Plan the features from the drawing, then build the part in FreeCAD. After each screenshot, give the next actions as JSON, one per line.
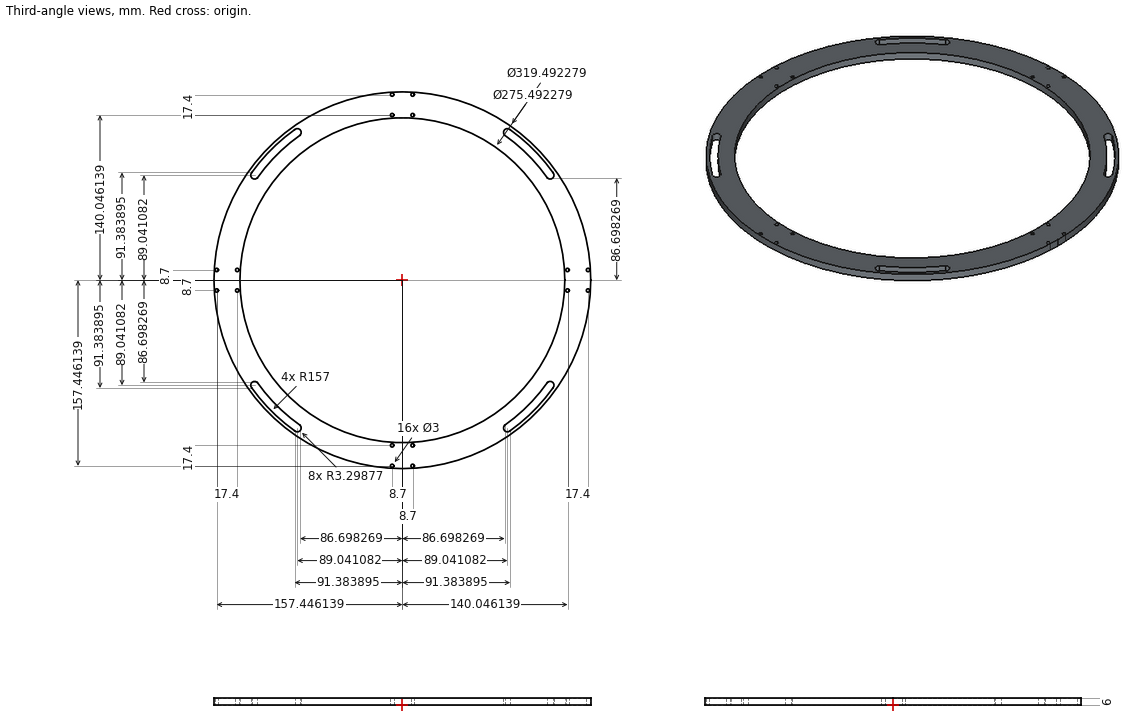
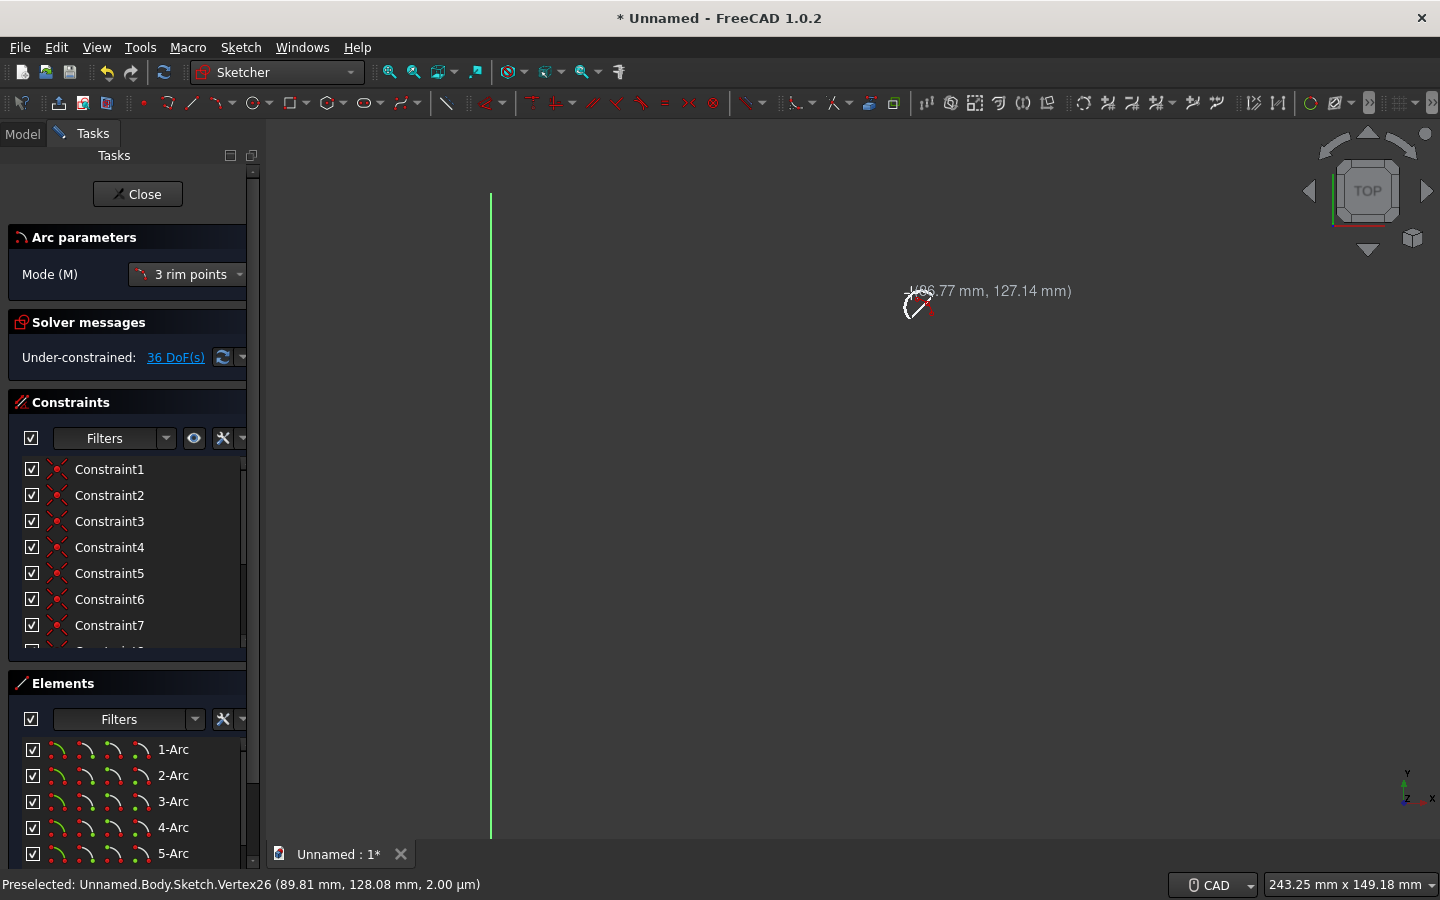
{"action": "left_click", "coordinate": [909, 293]}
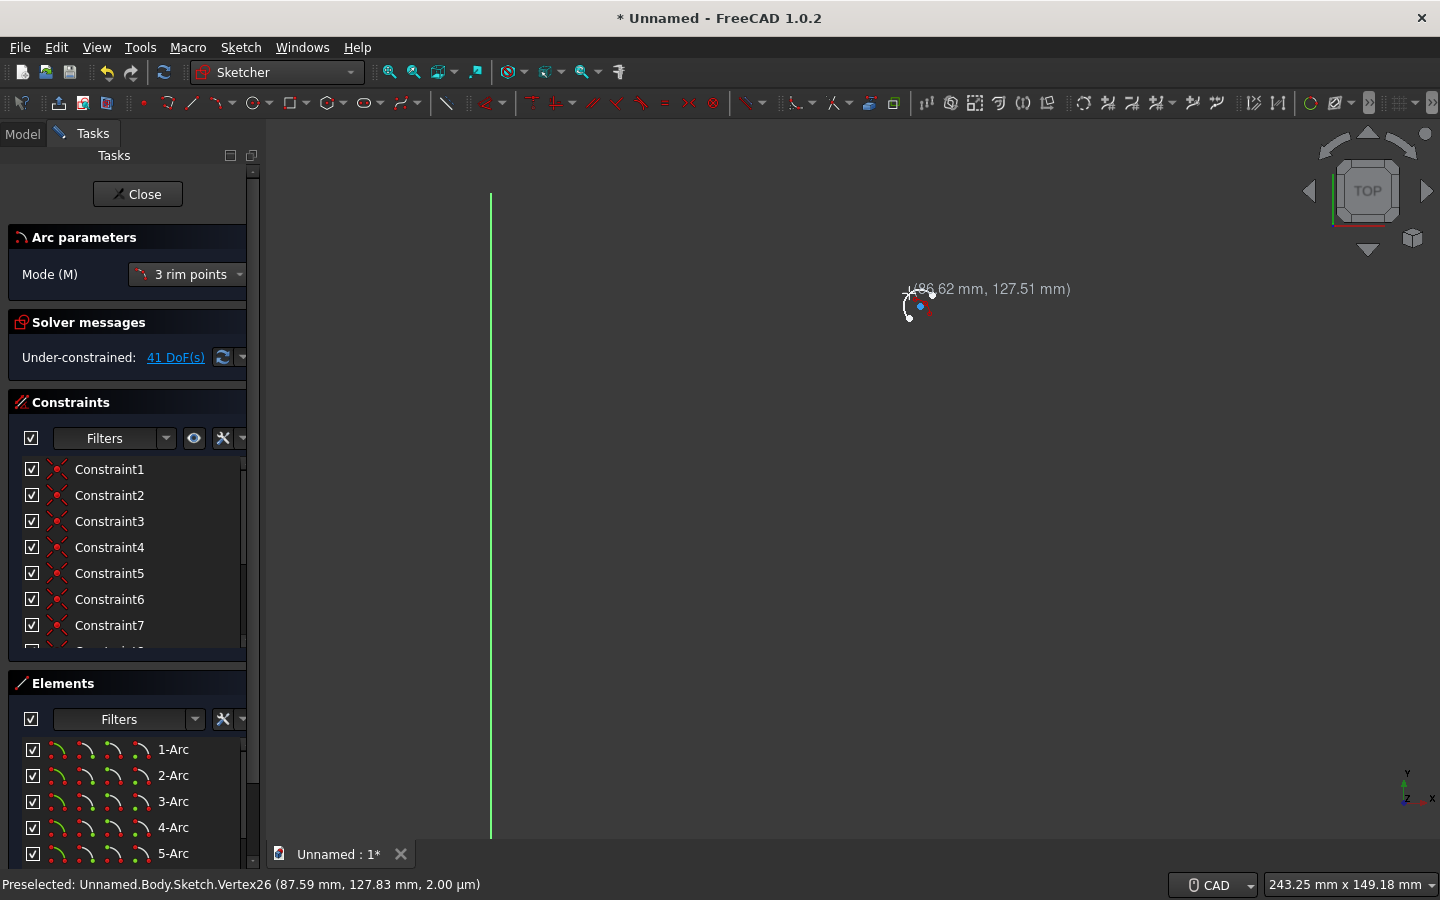
{"action": "left_click", "coordinate": [933, 296]}
{"action": "left_click", "coordinate": [1107, 468]}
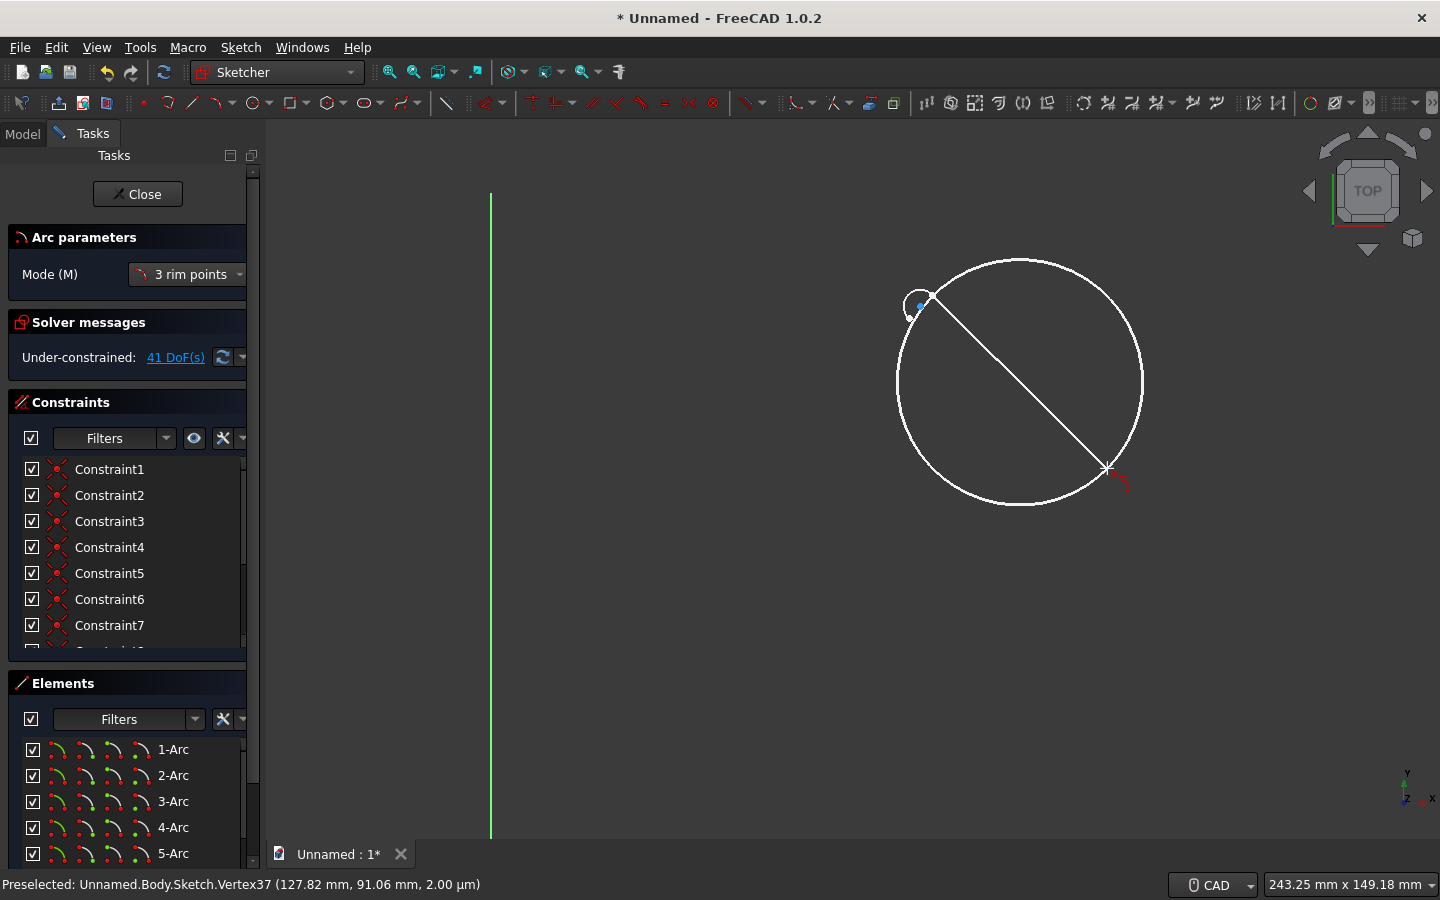
{"action": "scroll", "coordinate": [1027, 374], "scroll_direction": "up", "scroll_amount": 3}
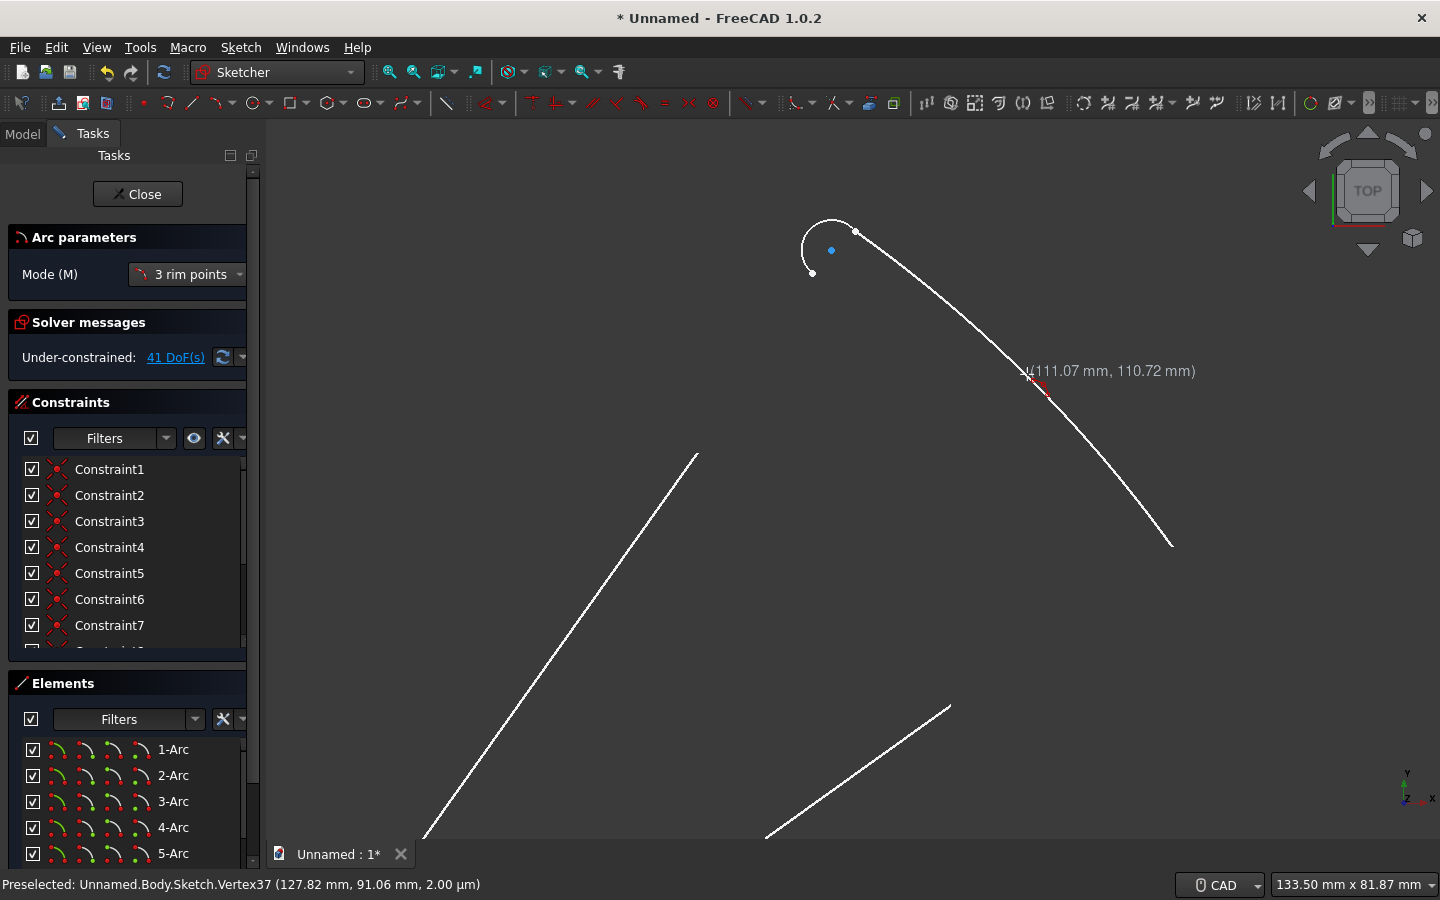
{"action": "left_click", "coordinate": [1026, 373]}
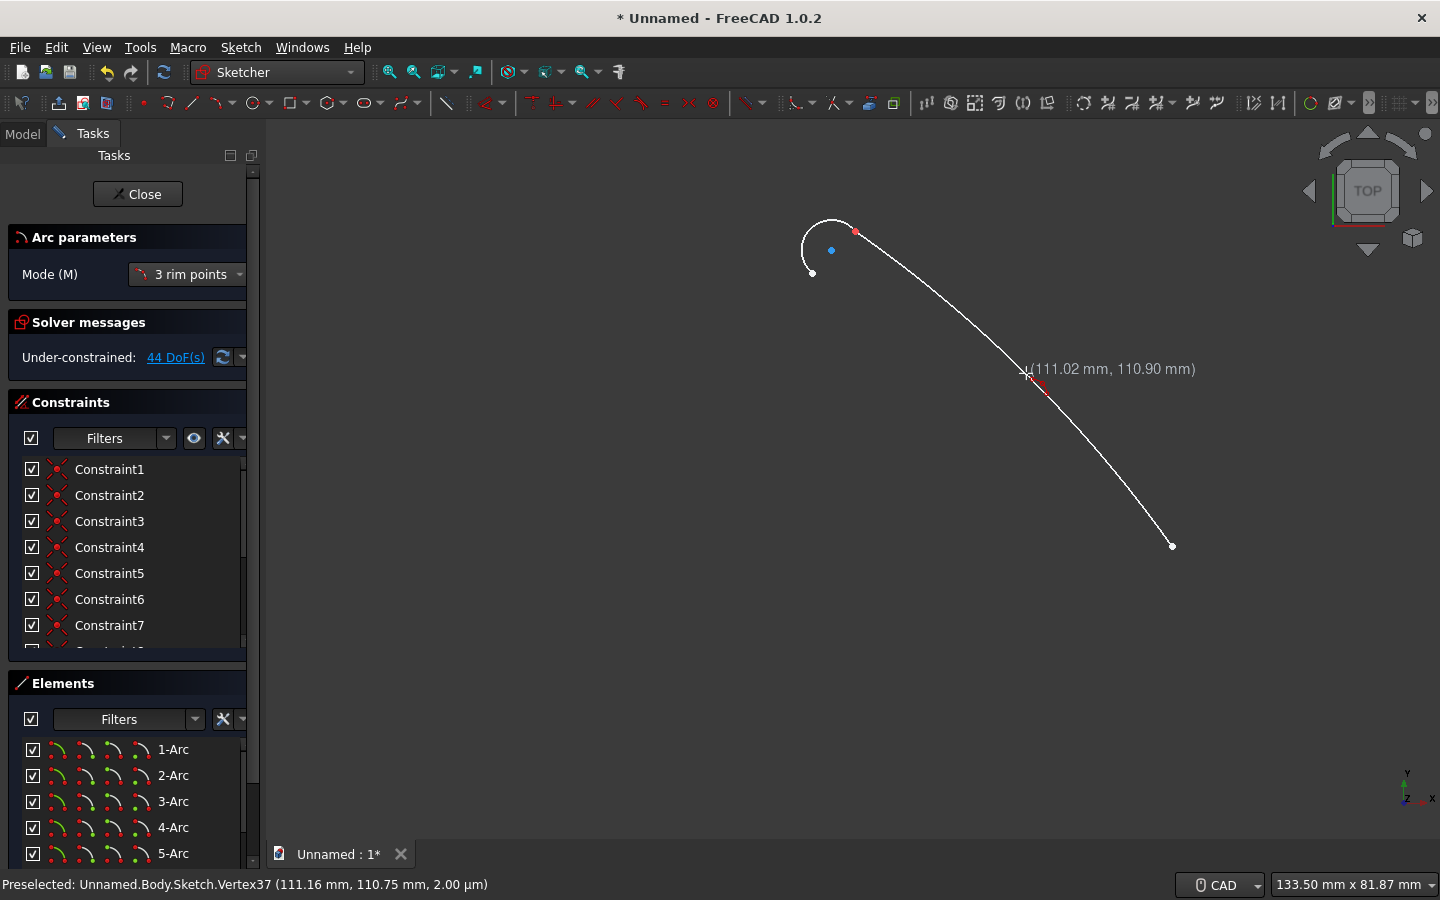
{"action": "scroll", "coordinate": [930, 307], "scroll_direction": "down", "scroll_amount": 9}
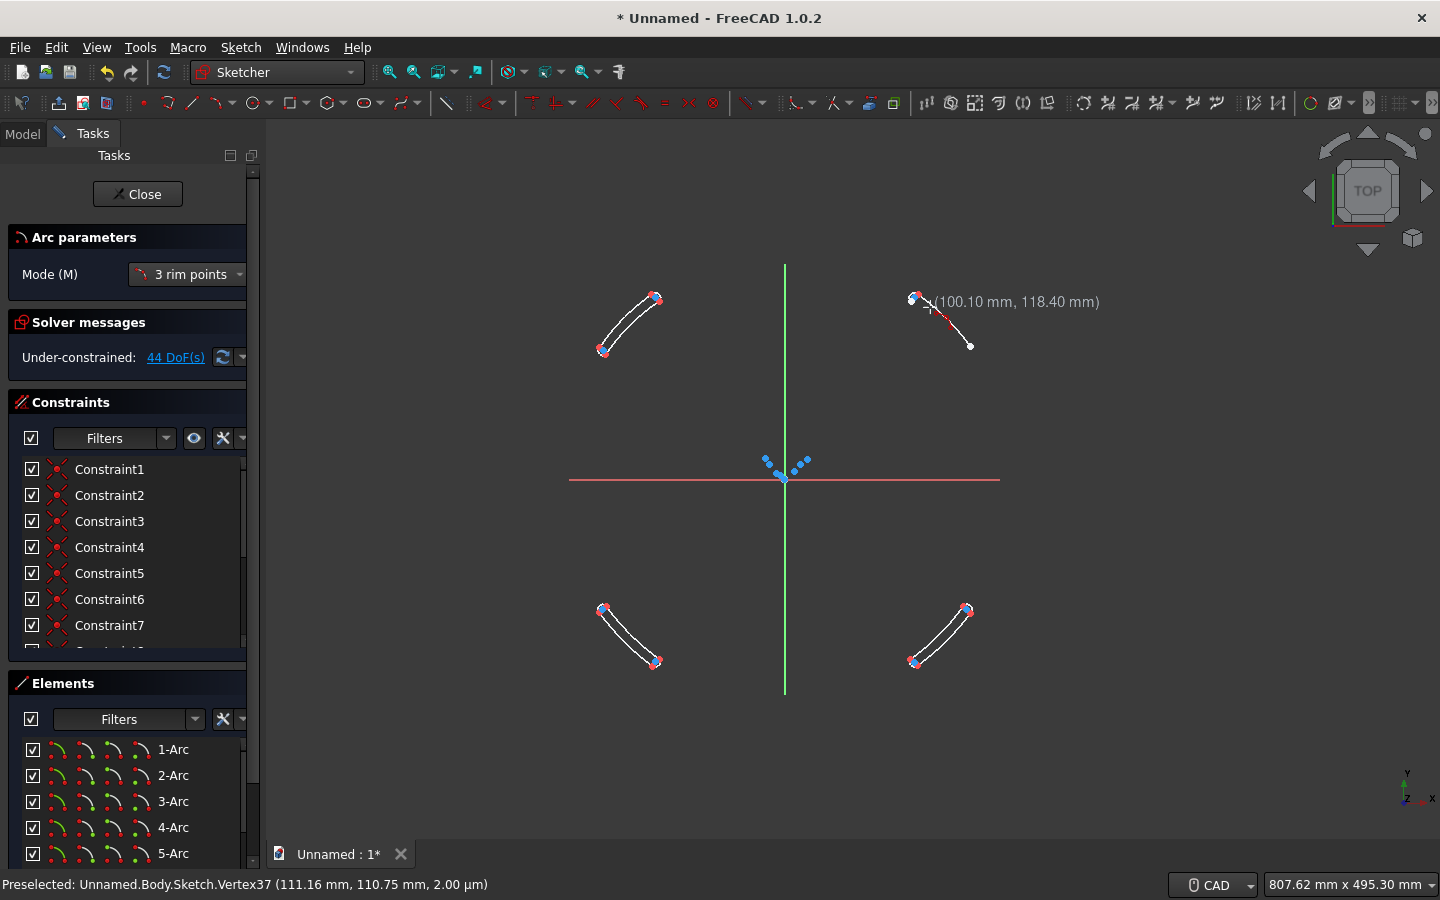
{"action": "left_click", "coordinate": [971, 347]}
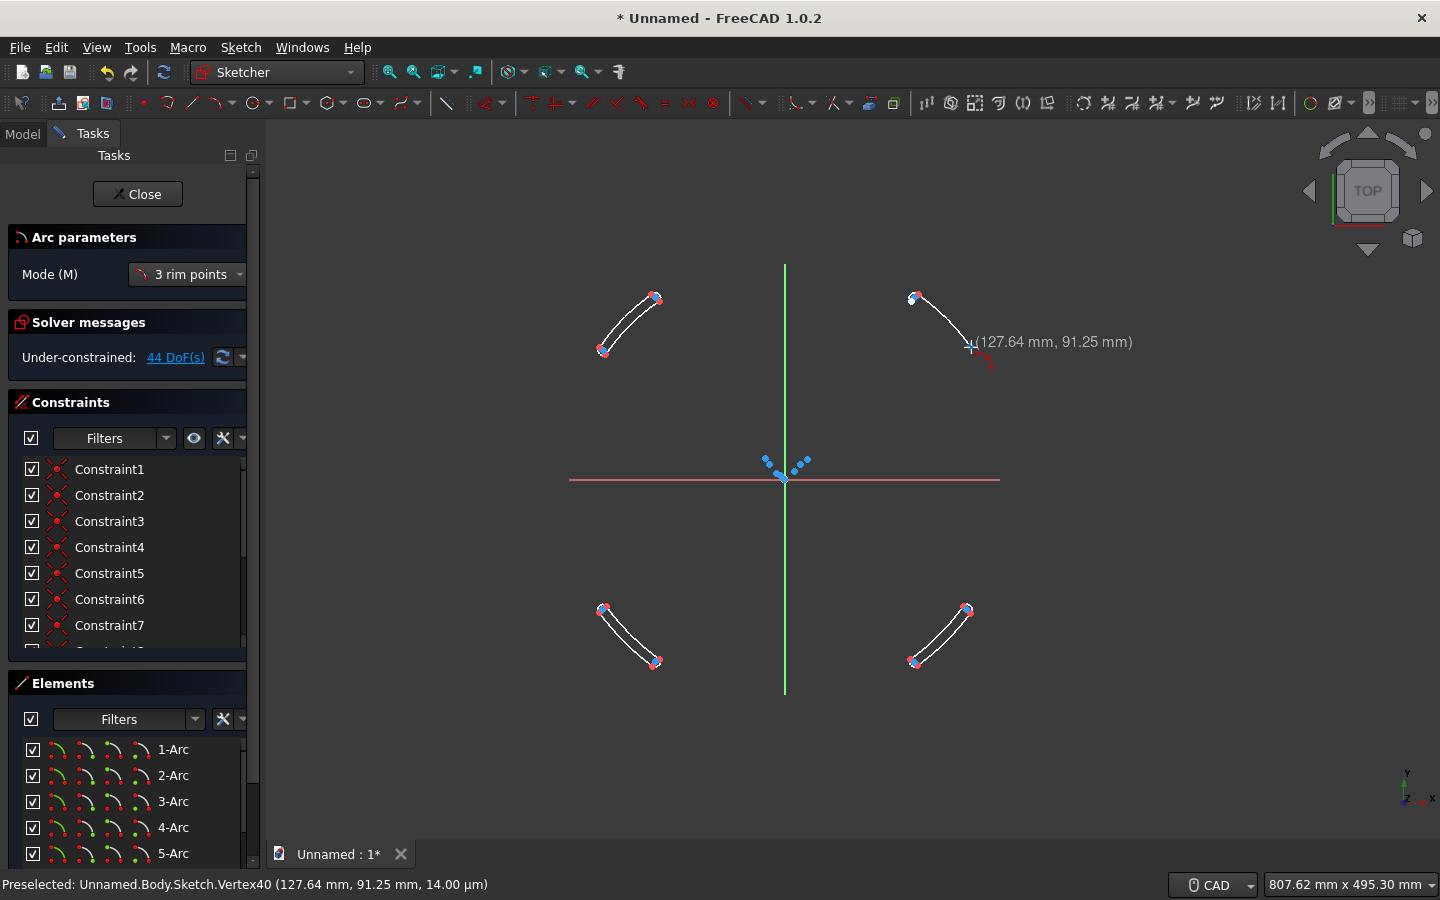
{"action": "scroll", "coordinate": [964, 353], "scroll_direction": "up", "scroll_amount": 3}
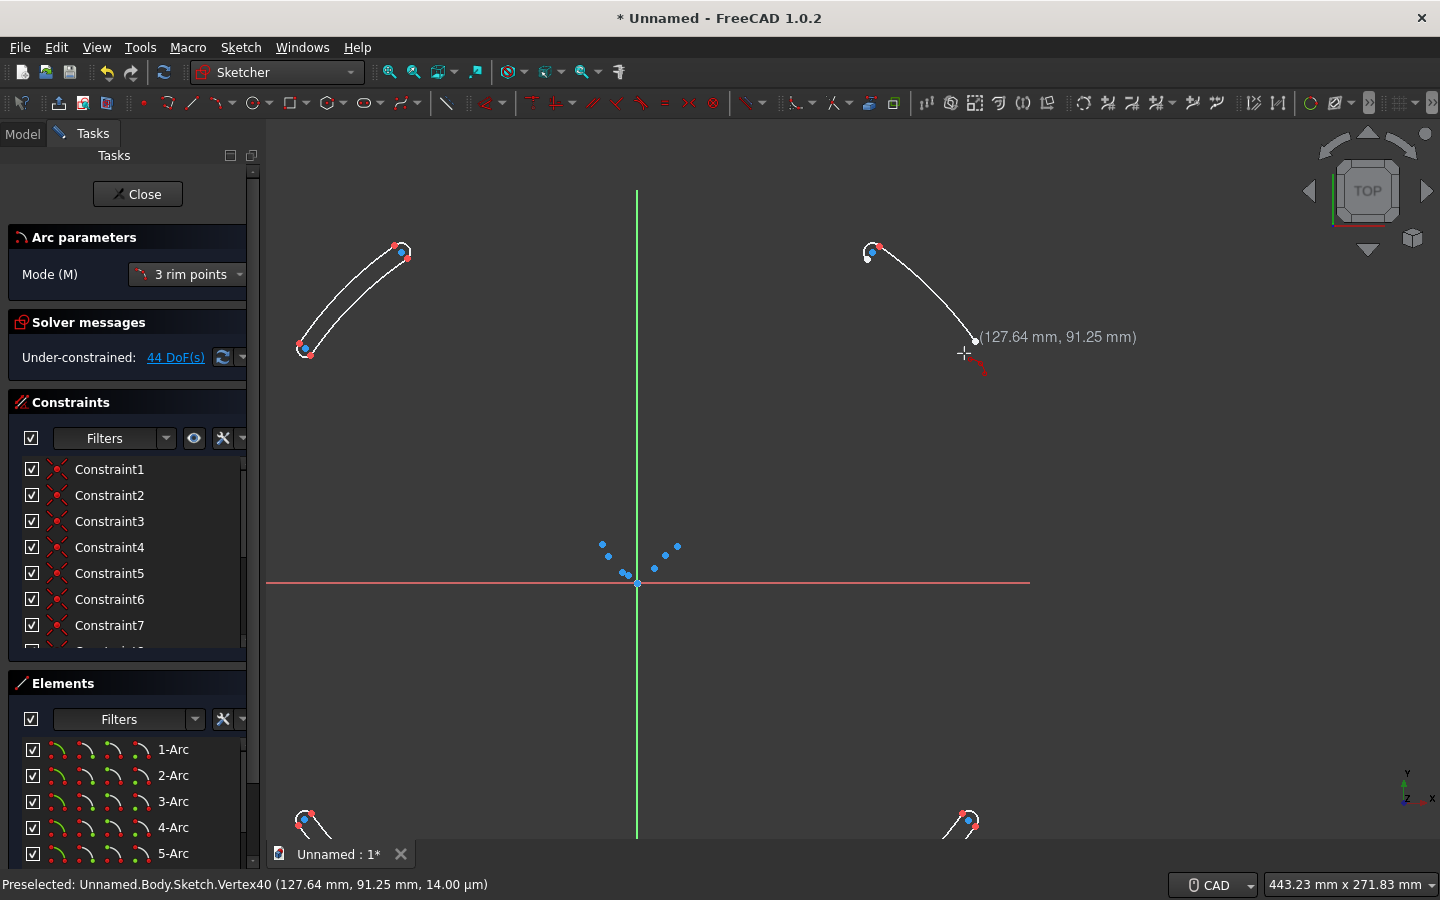
{"action": "left_click", "coordinate": [963, 354]}